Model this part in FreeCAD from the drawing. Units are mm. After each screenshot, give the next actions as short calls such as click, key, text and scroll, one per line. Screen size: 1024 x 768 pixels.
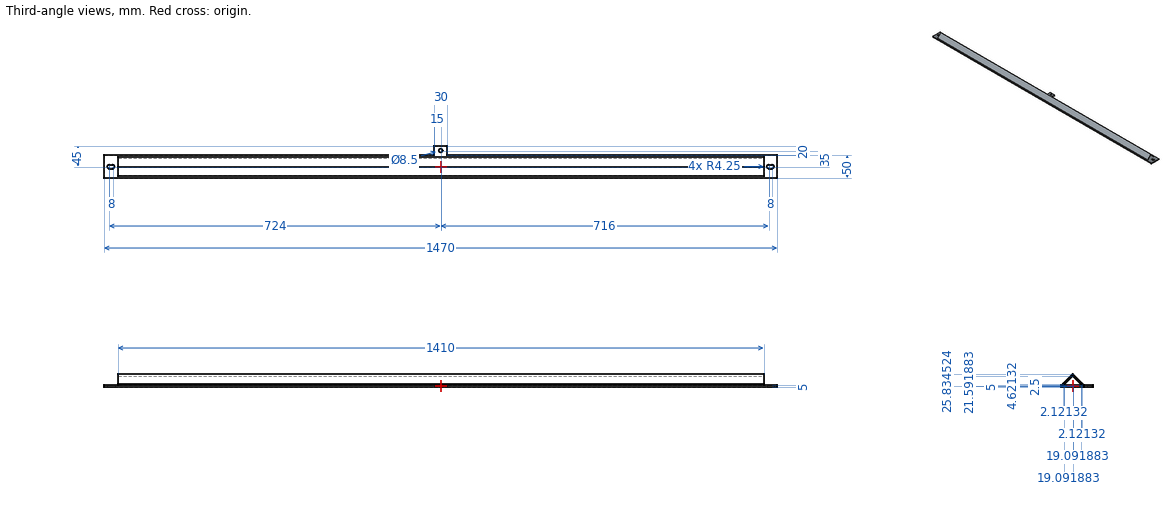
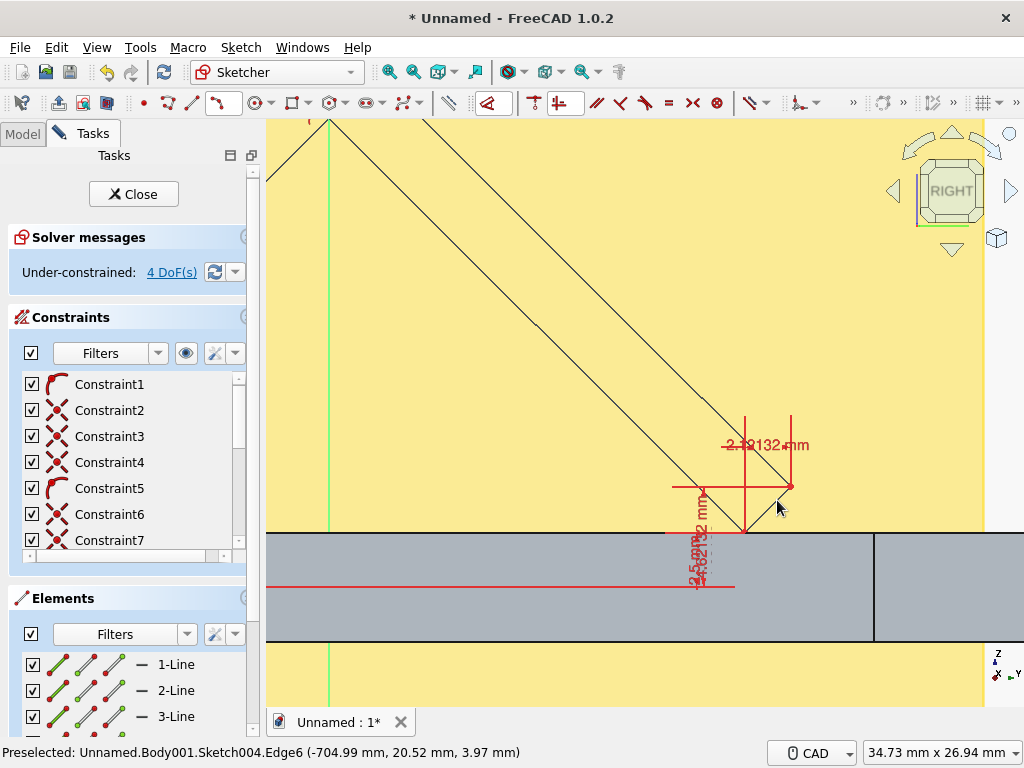
click(745, 533)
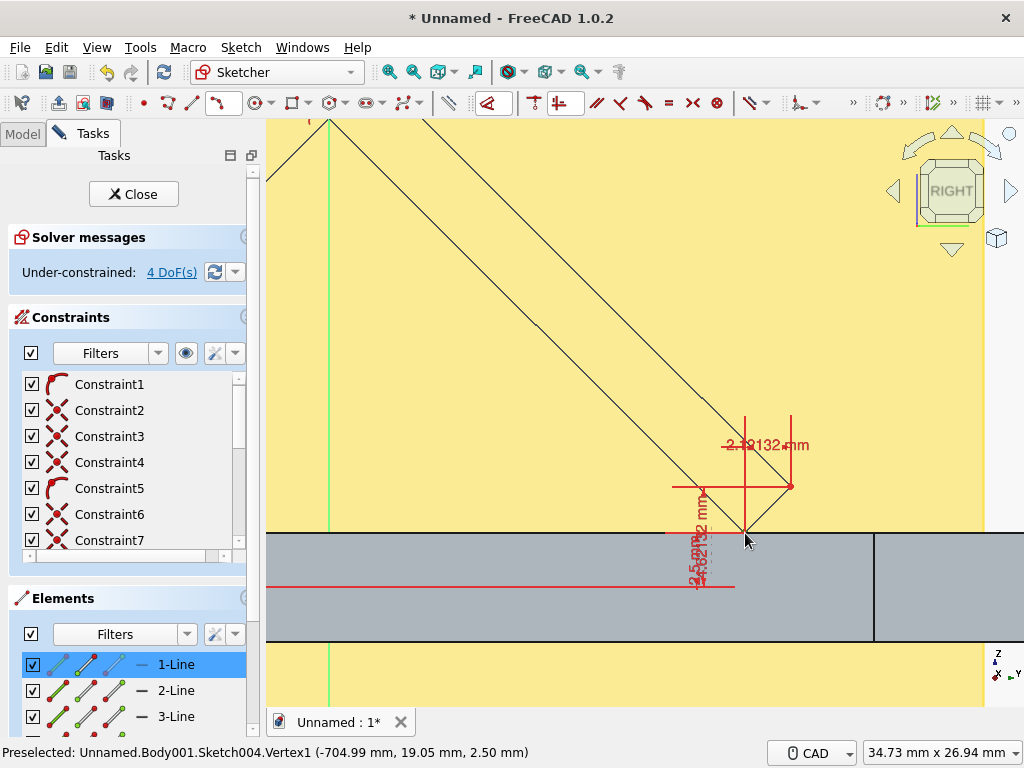
key(l)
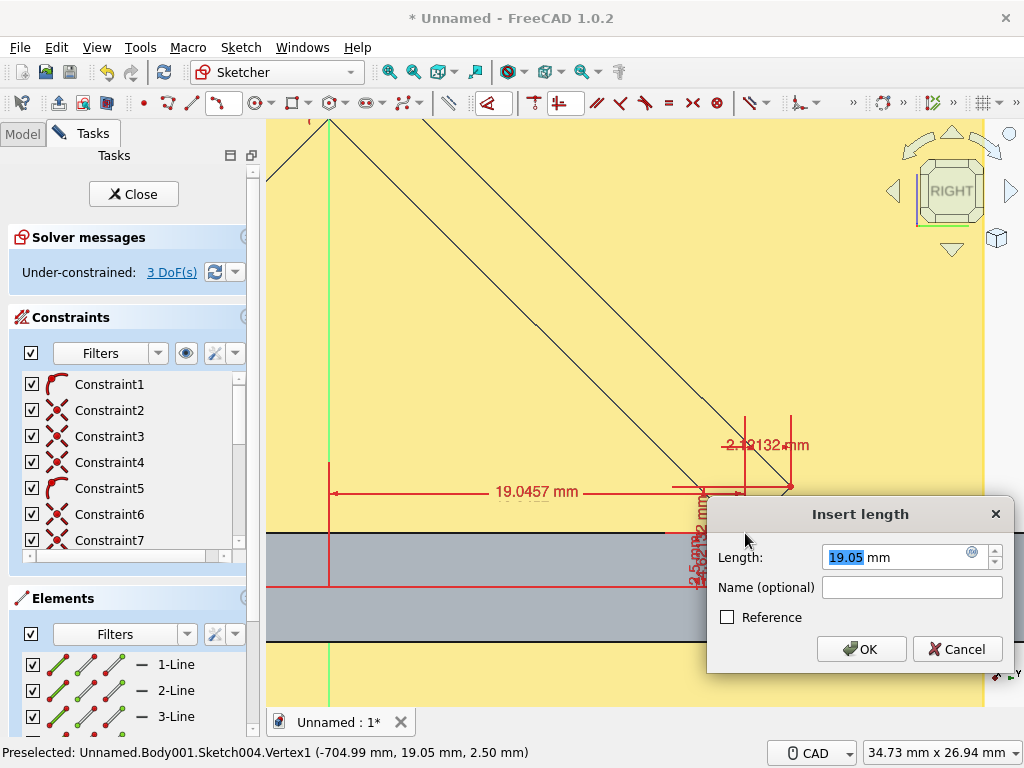
text(19.091883)
key(Return)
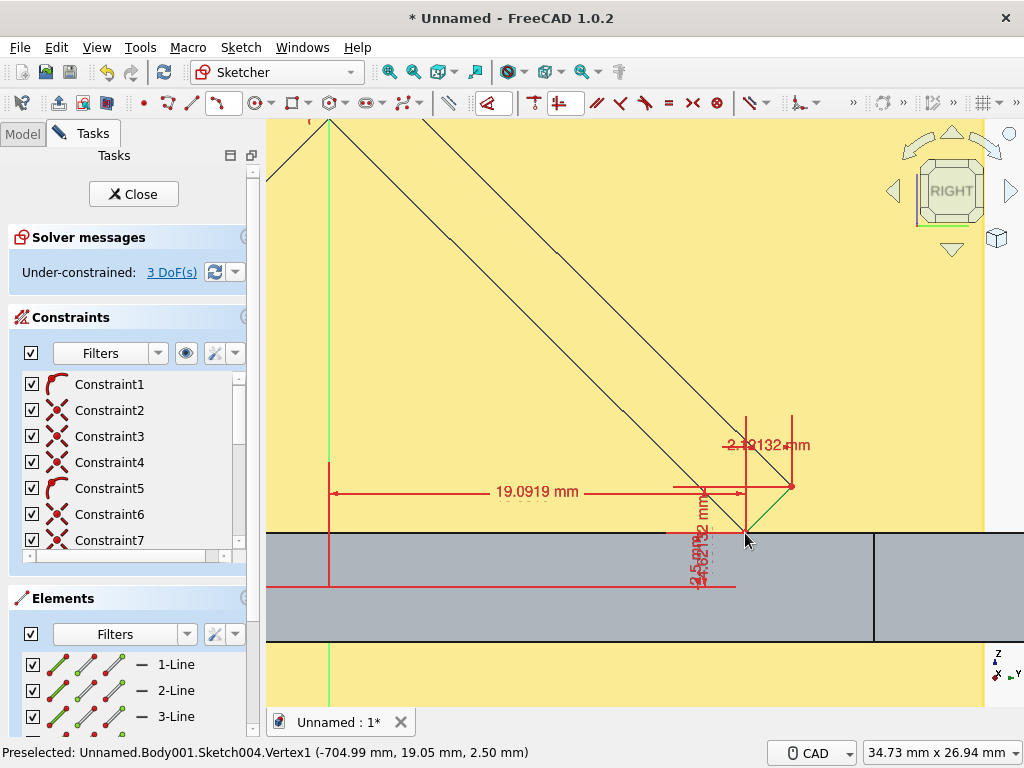
scroll(779, 501, down, 4)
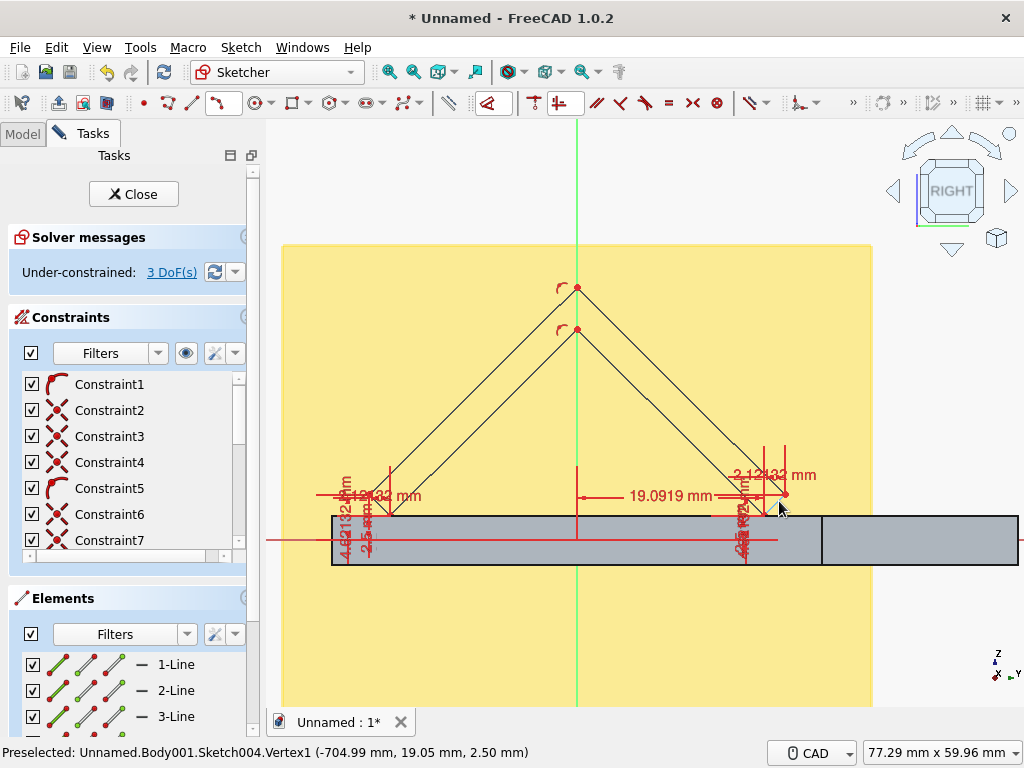
click(577, 330)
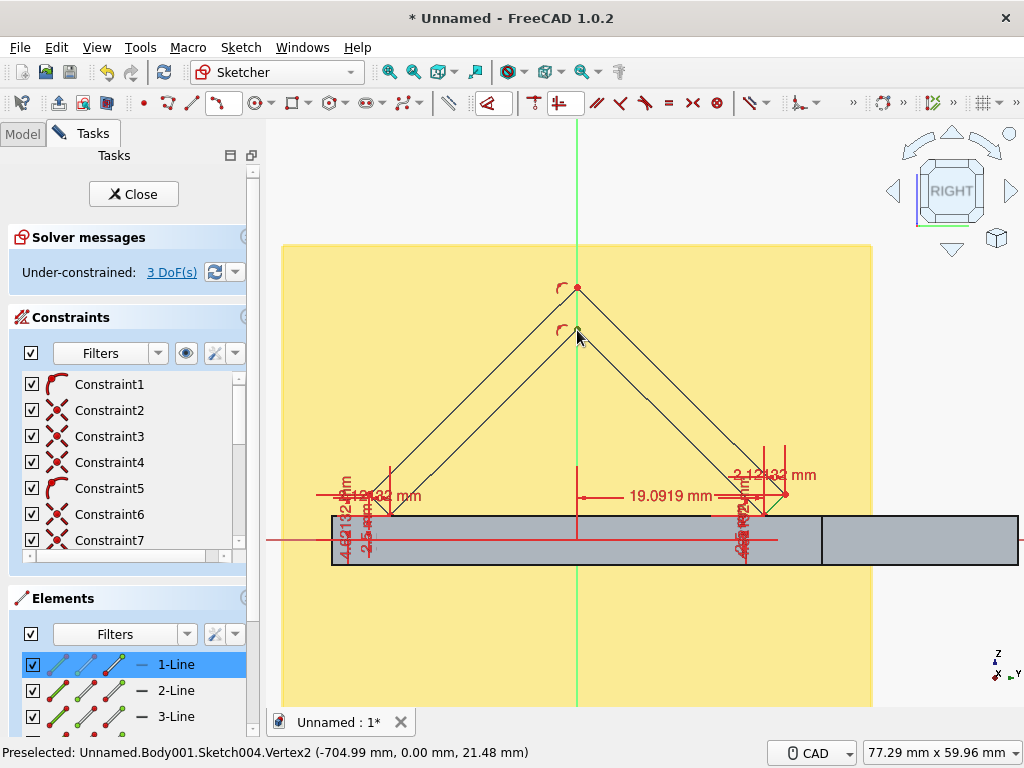
click(506, 104)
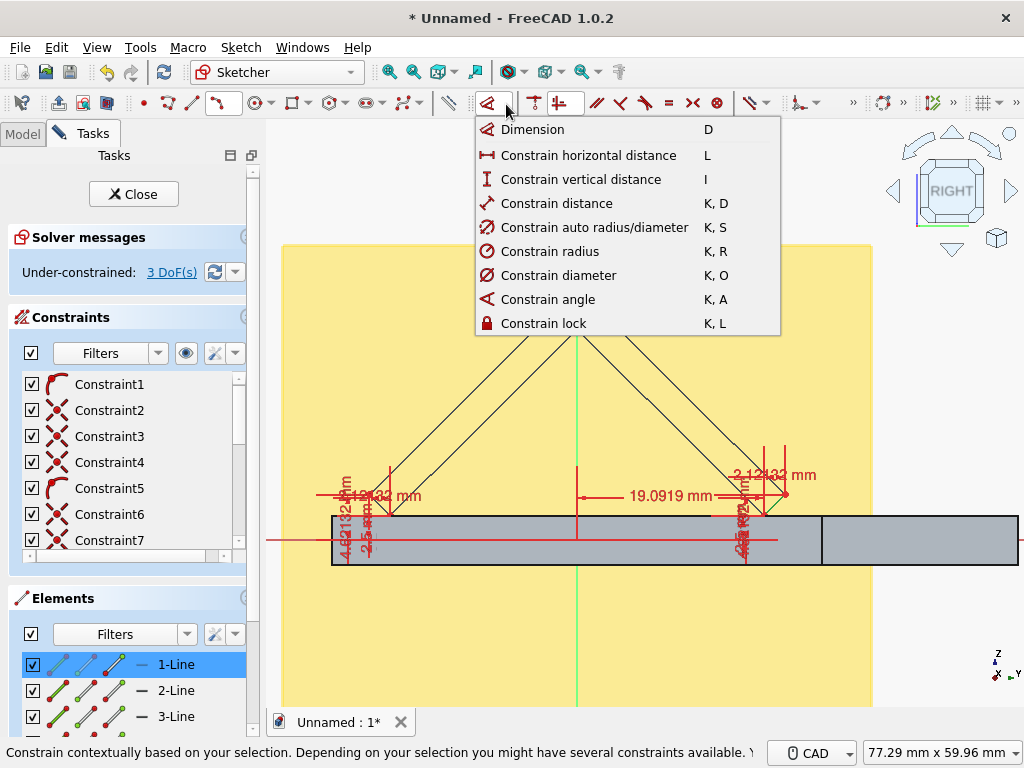
click(628, 179)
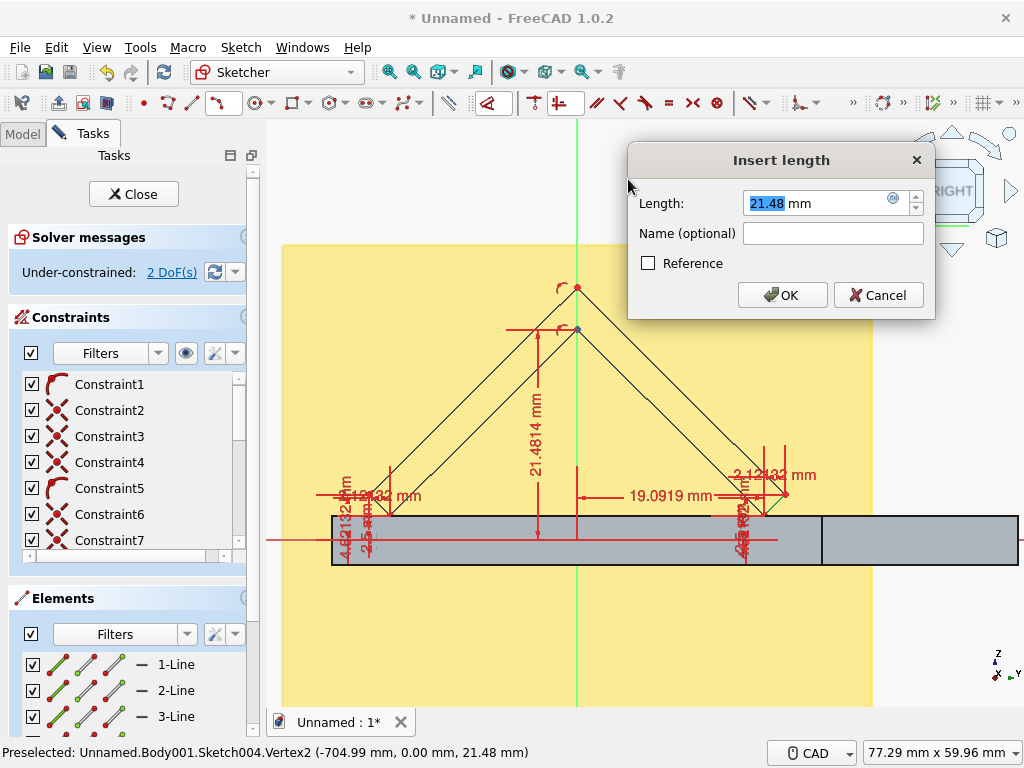
text(21.591883)
key(Return)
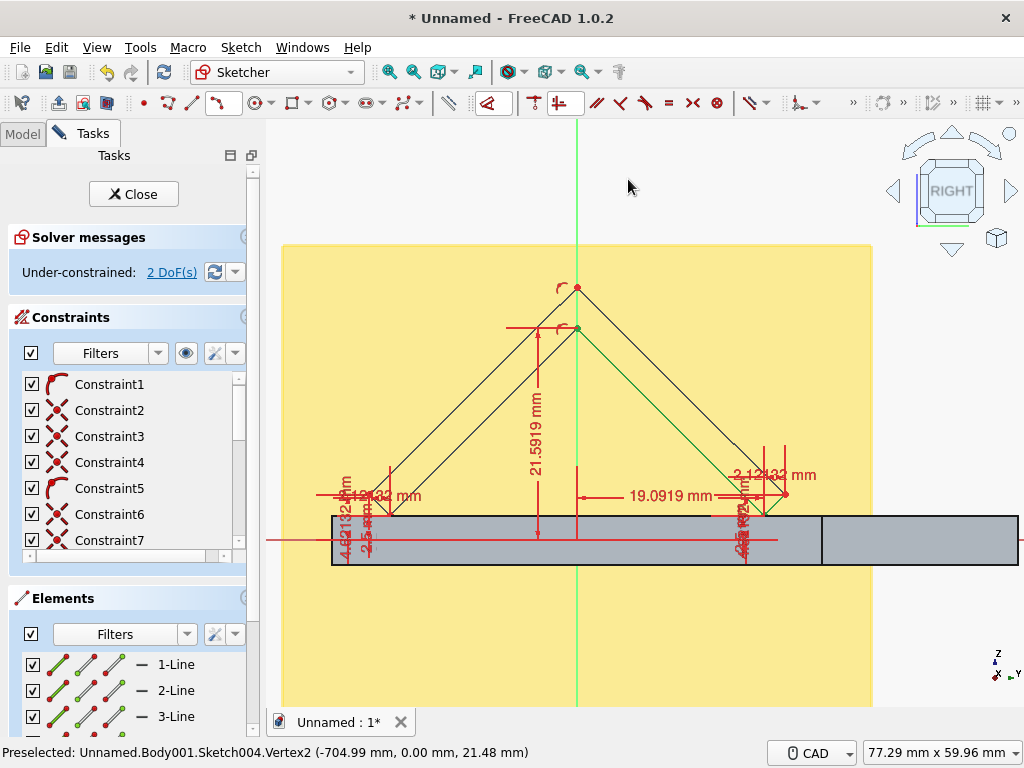
click(390, 516)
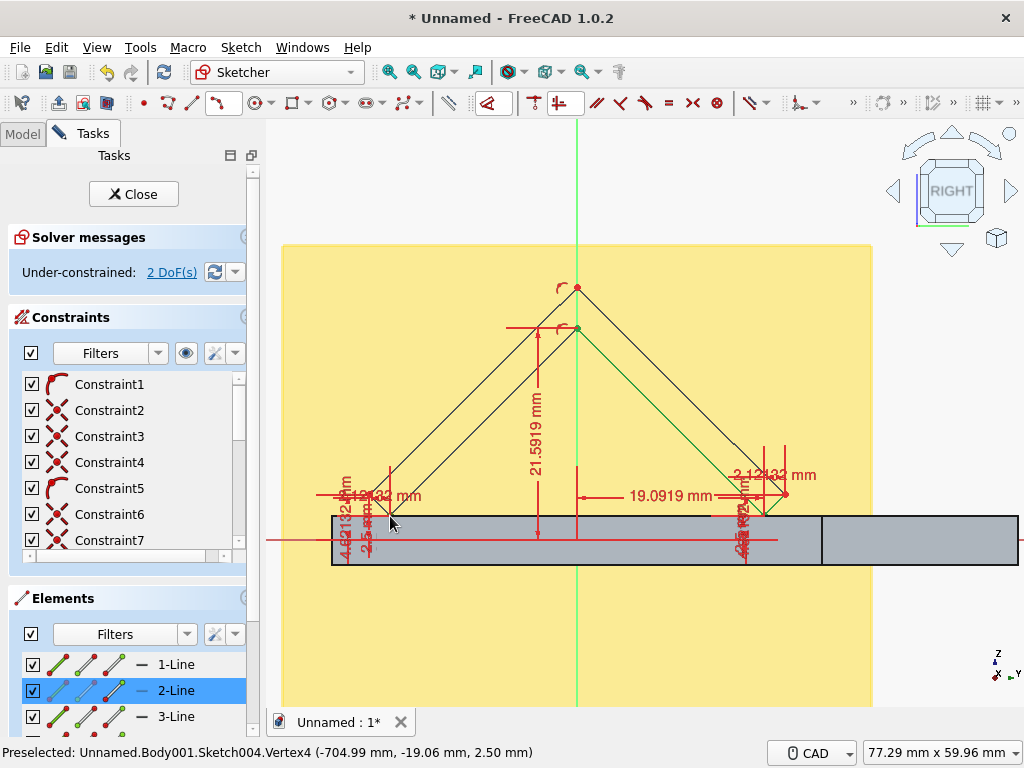
click(506, 104)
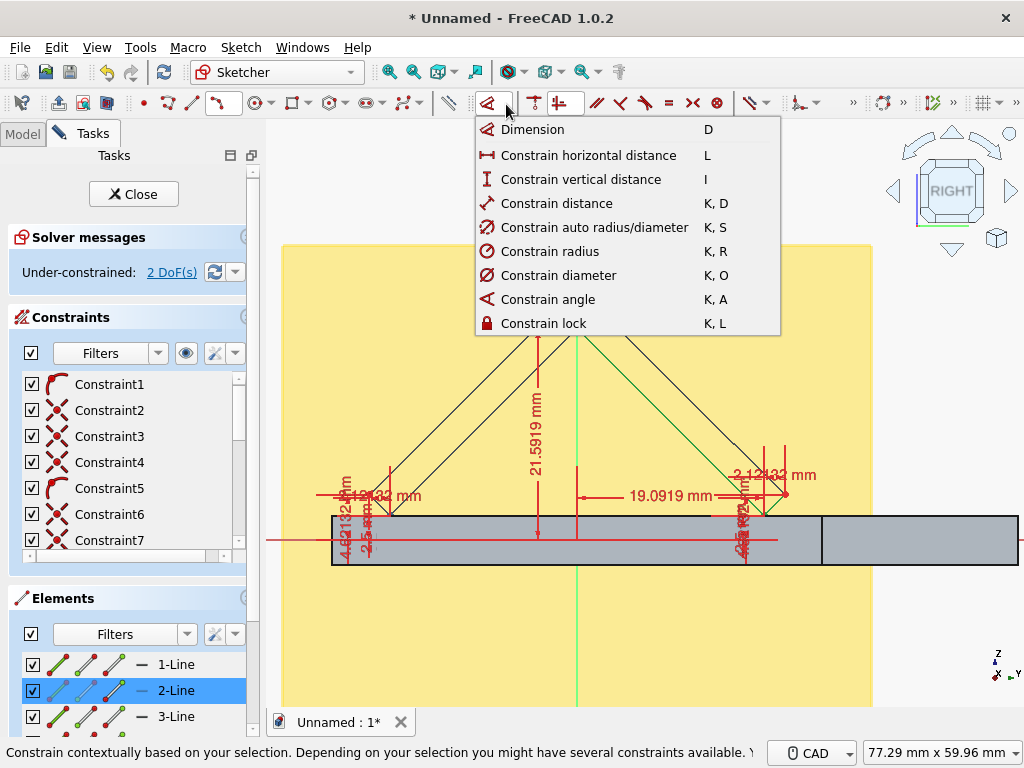
click(628, 155)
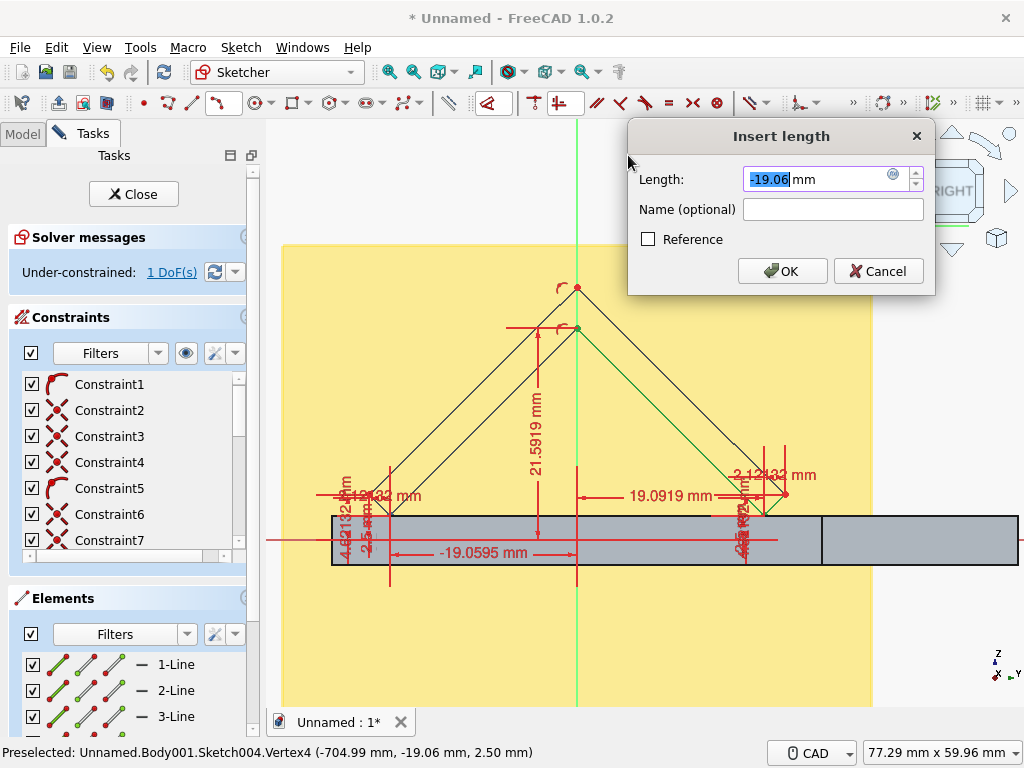
text(-19.091883)
key(Return)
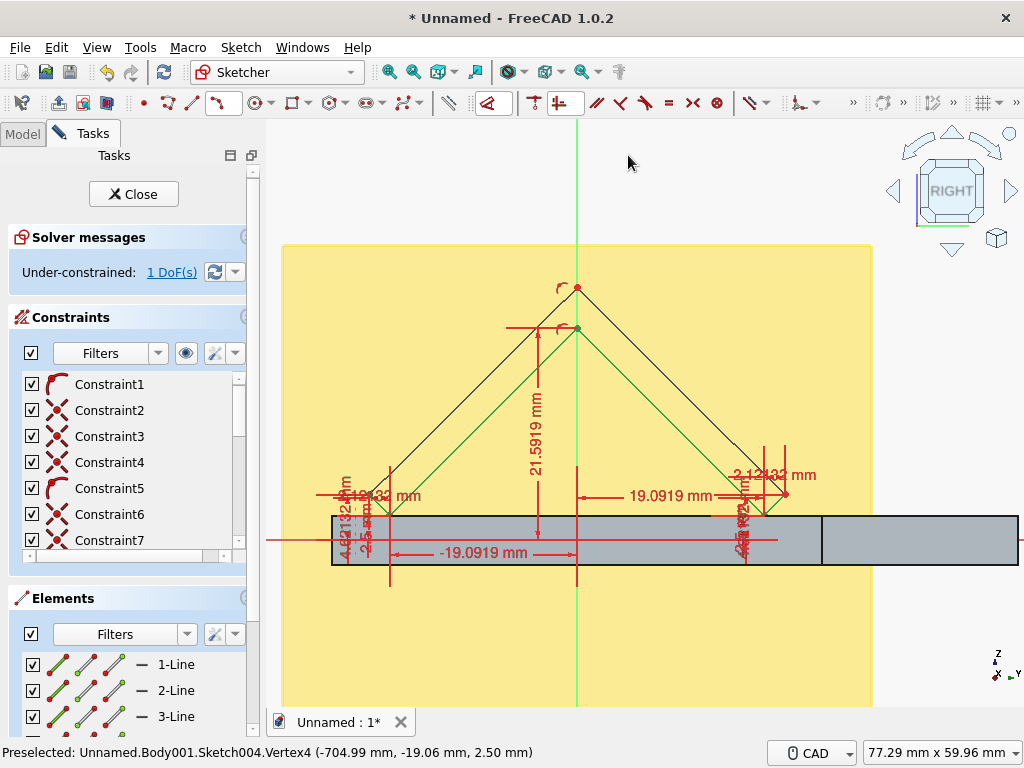
click(577, 288)